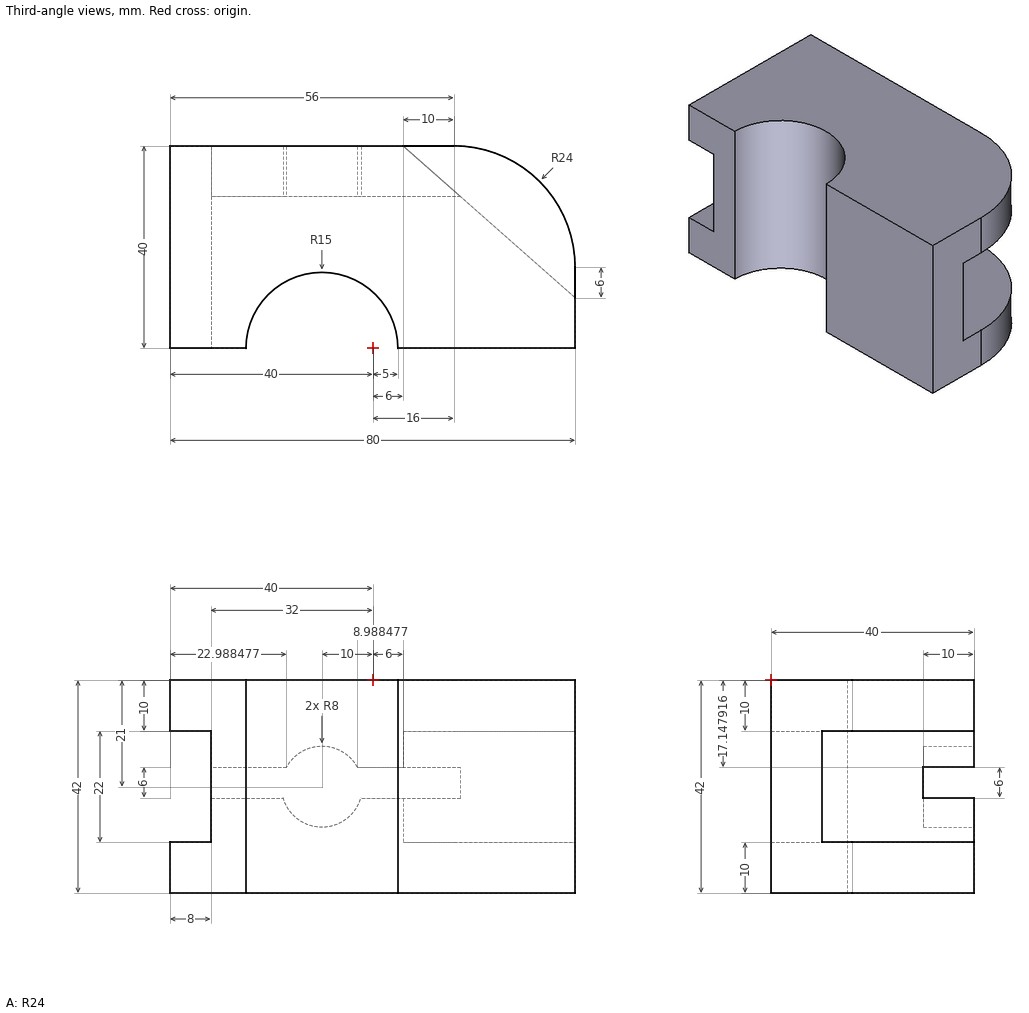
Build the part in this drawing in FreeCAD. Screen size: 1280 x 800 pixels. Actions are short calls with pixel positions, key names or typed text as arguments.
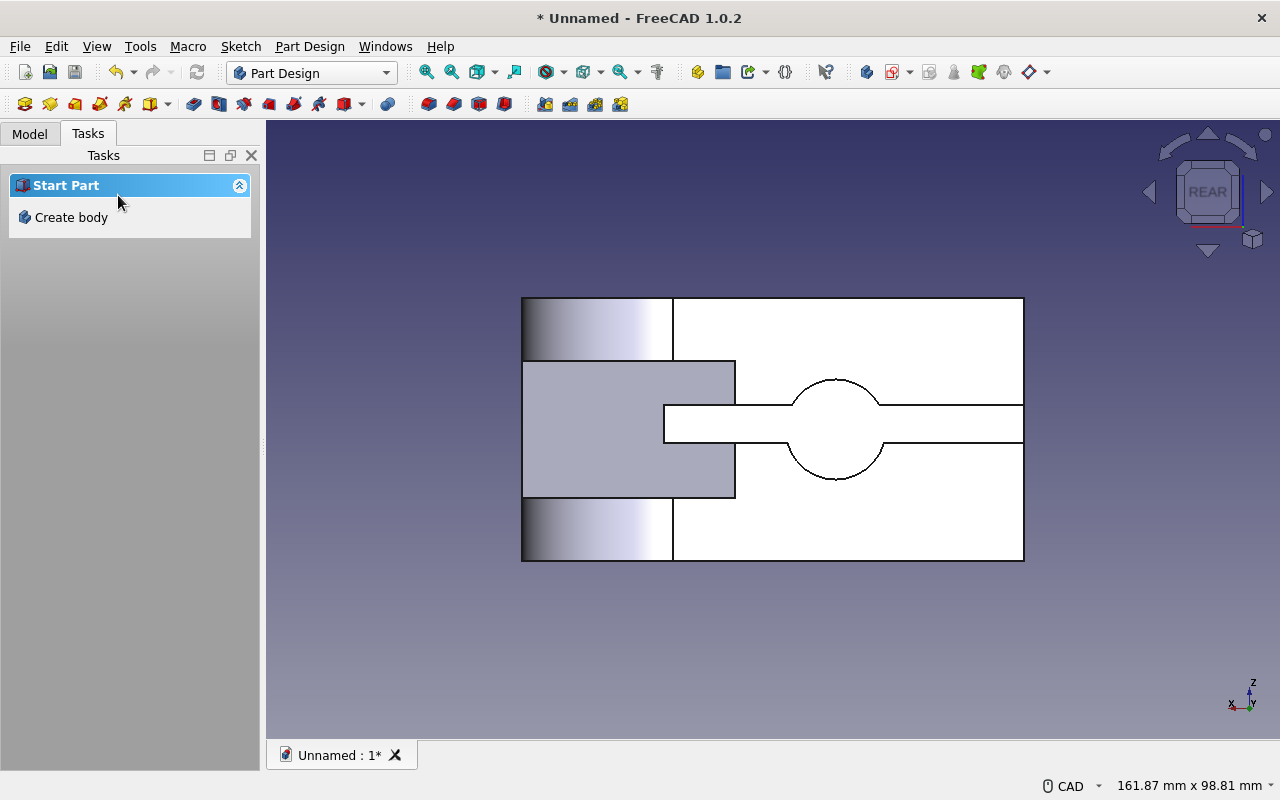
click(948, 501)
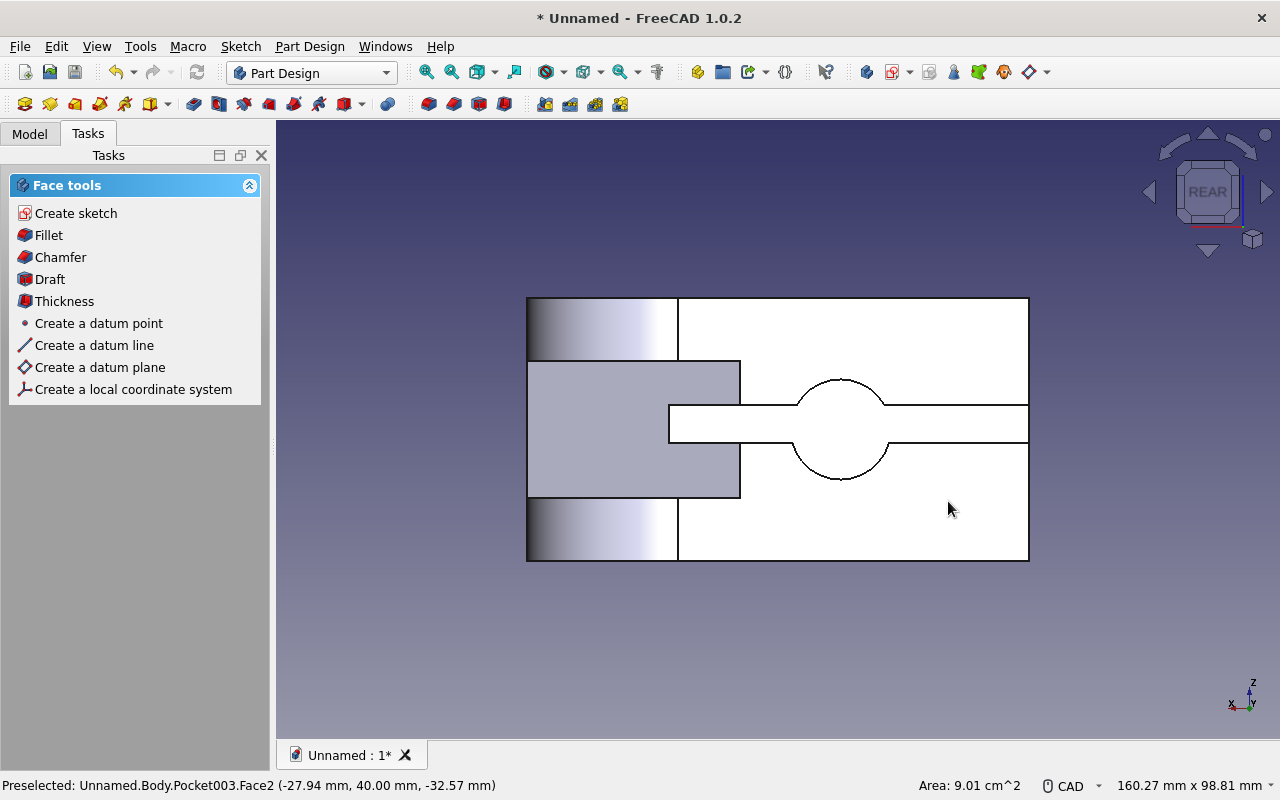
click(892, 72)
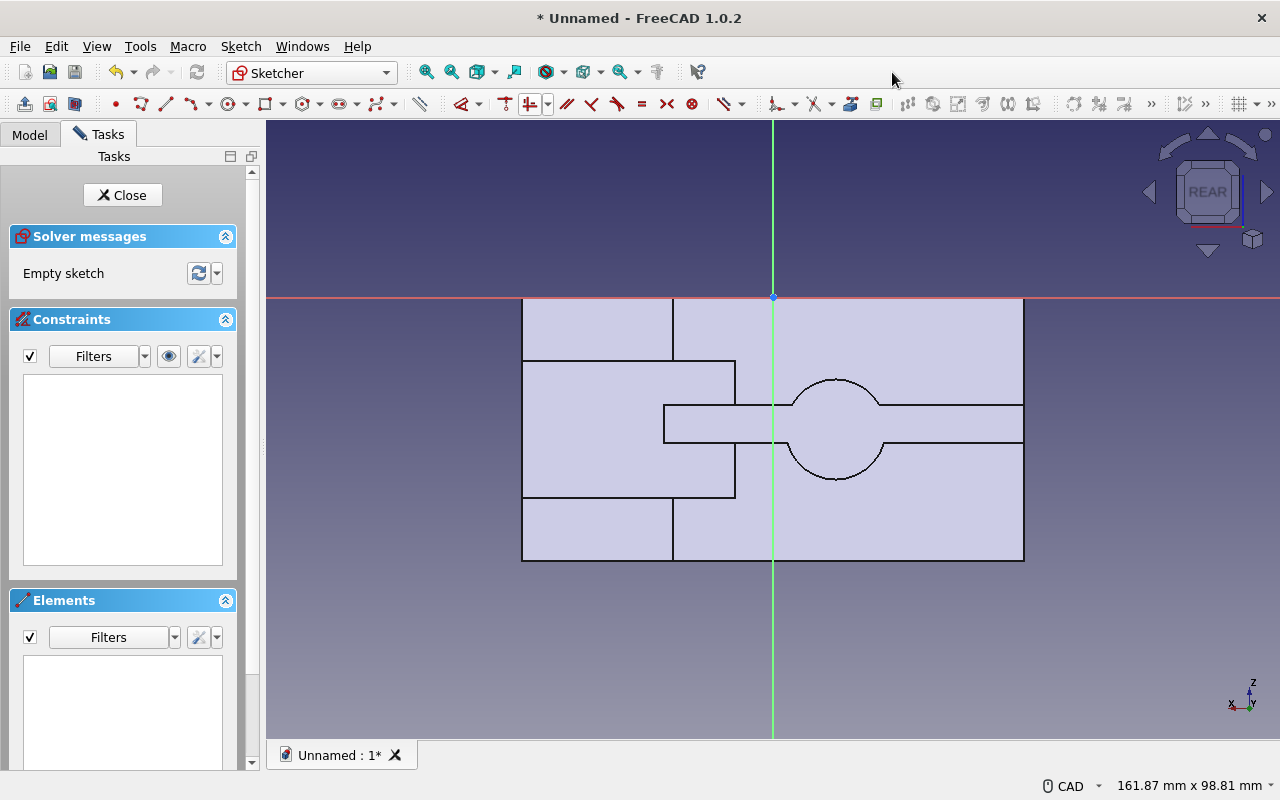
scroll(1115, 360, up, 3)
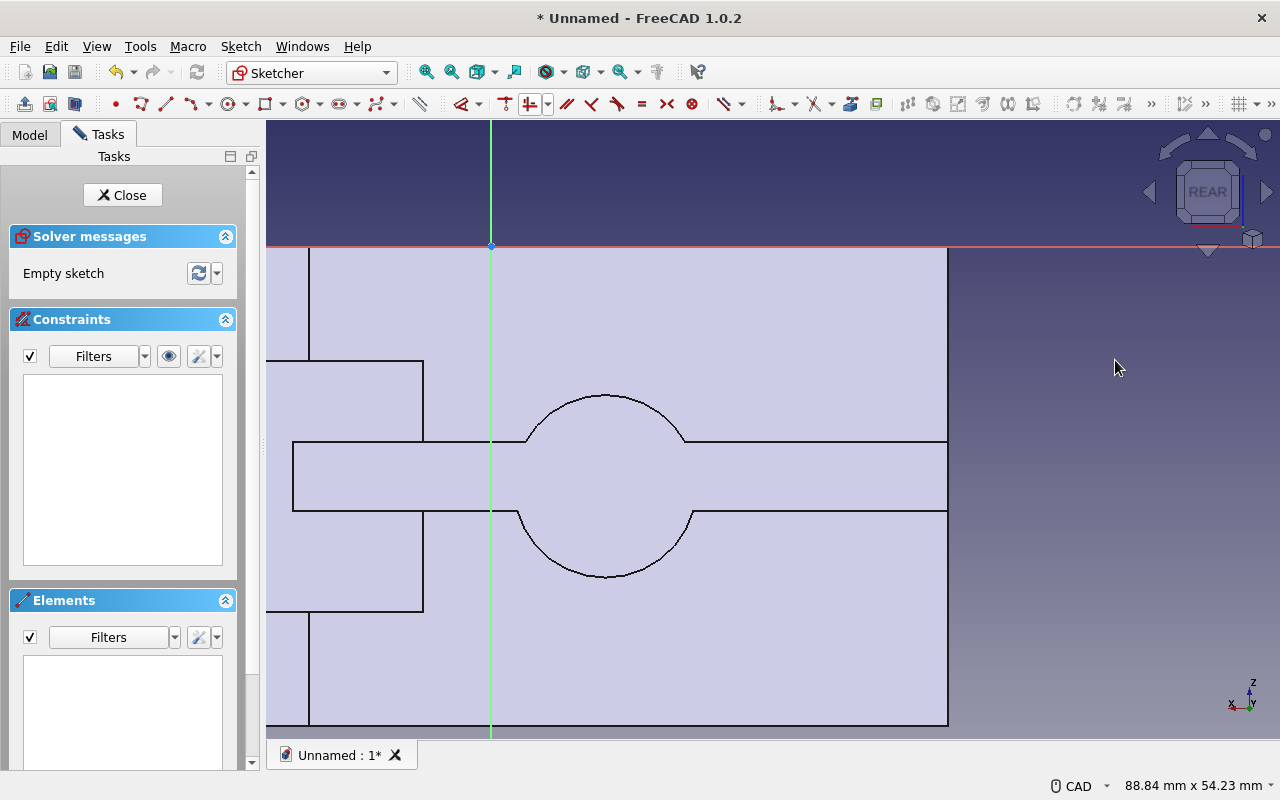
key(g)
key(r)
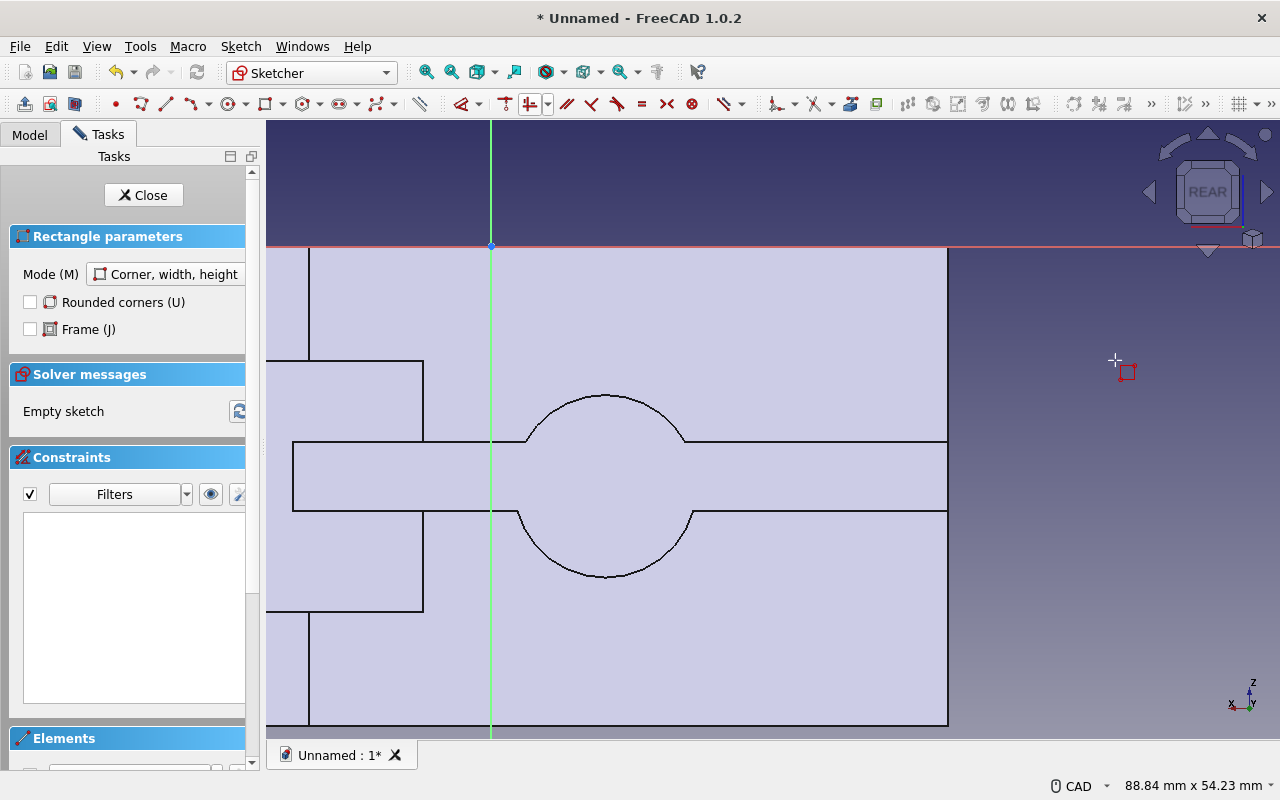
click(856, 361)
move(948, 612)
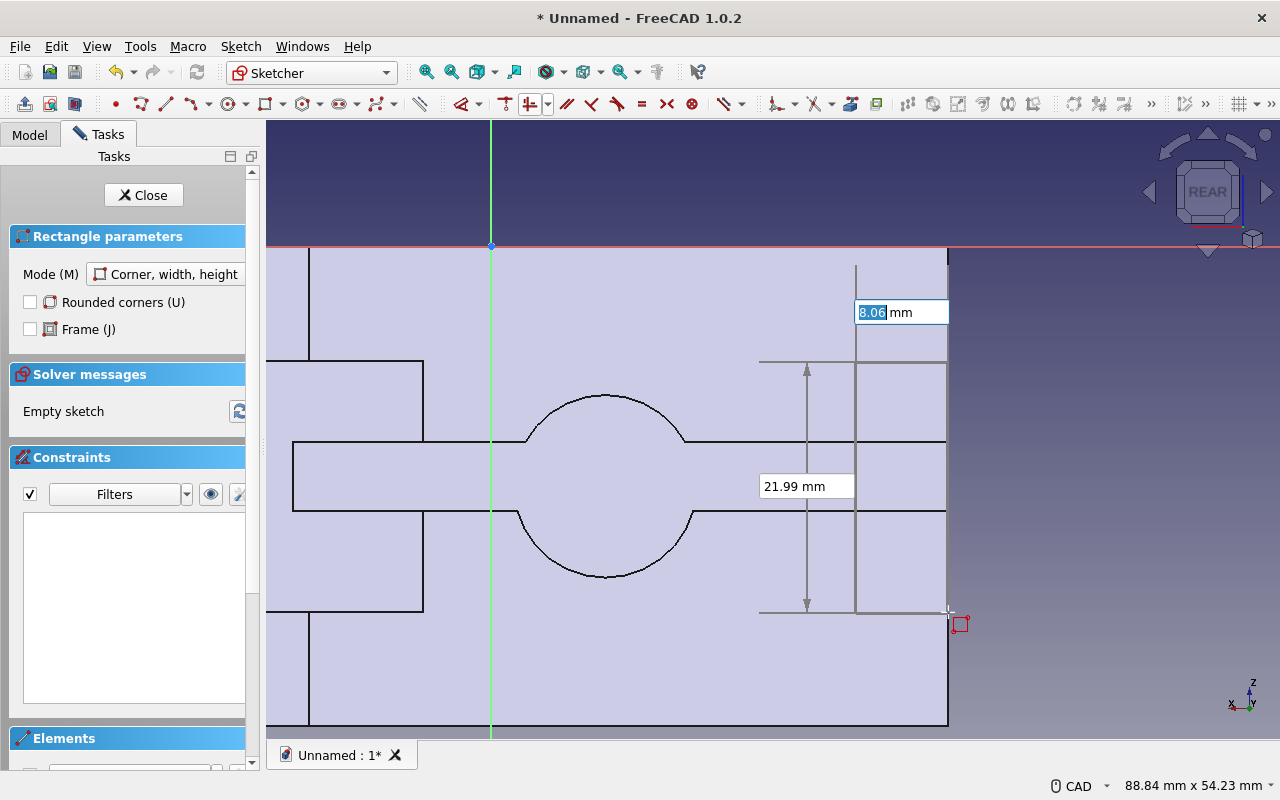
text(8)
key(Tab)
text(22)
key(Return)
key(Escape)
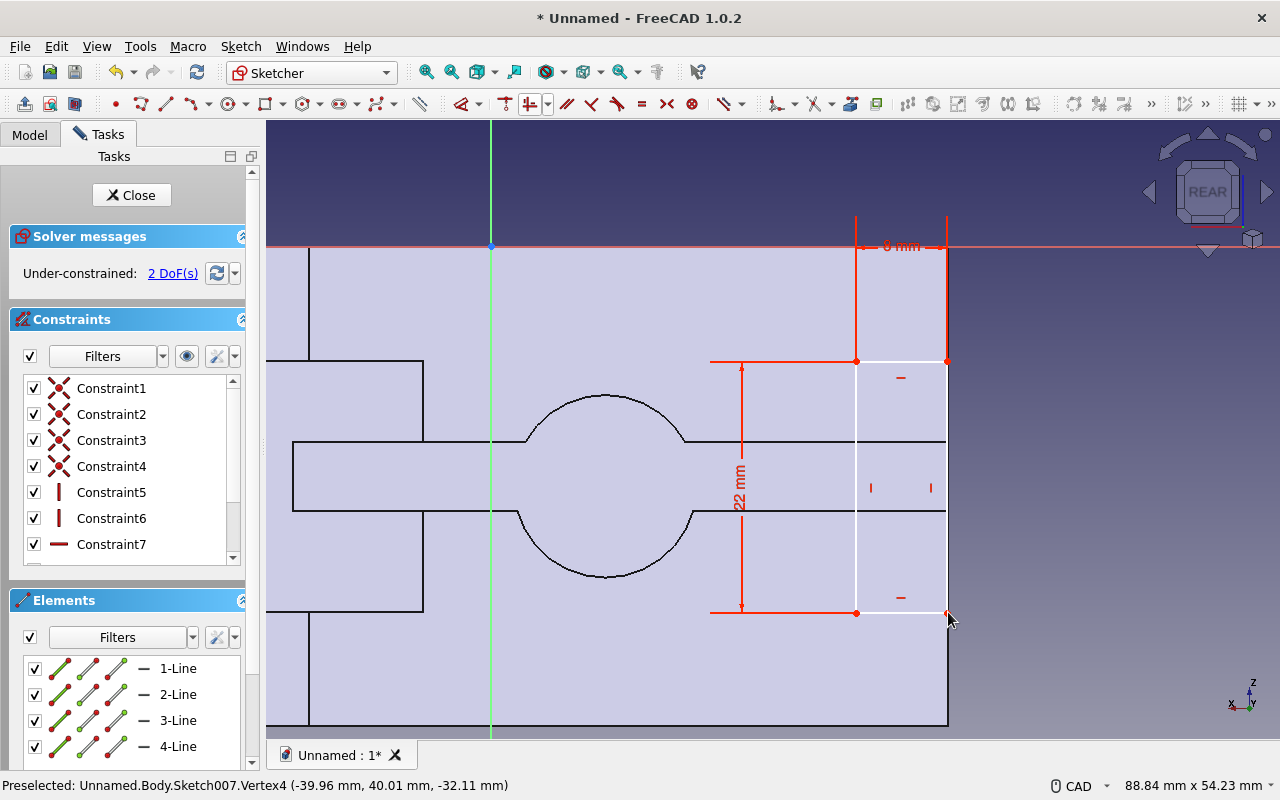
key(d)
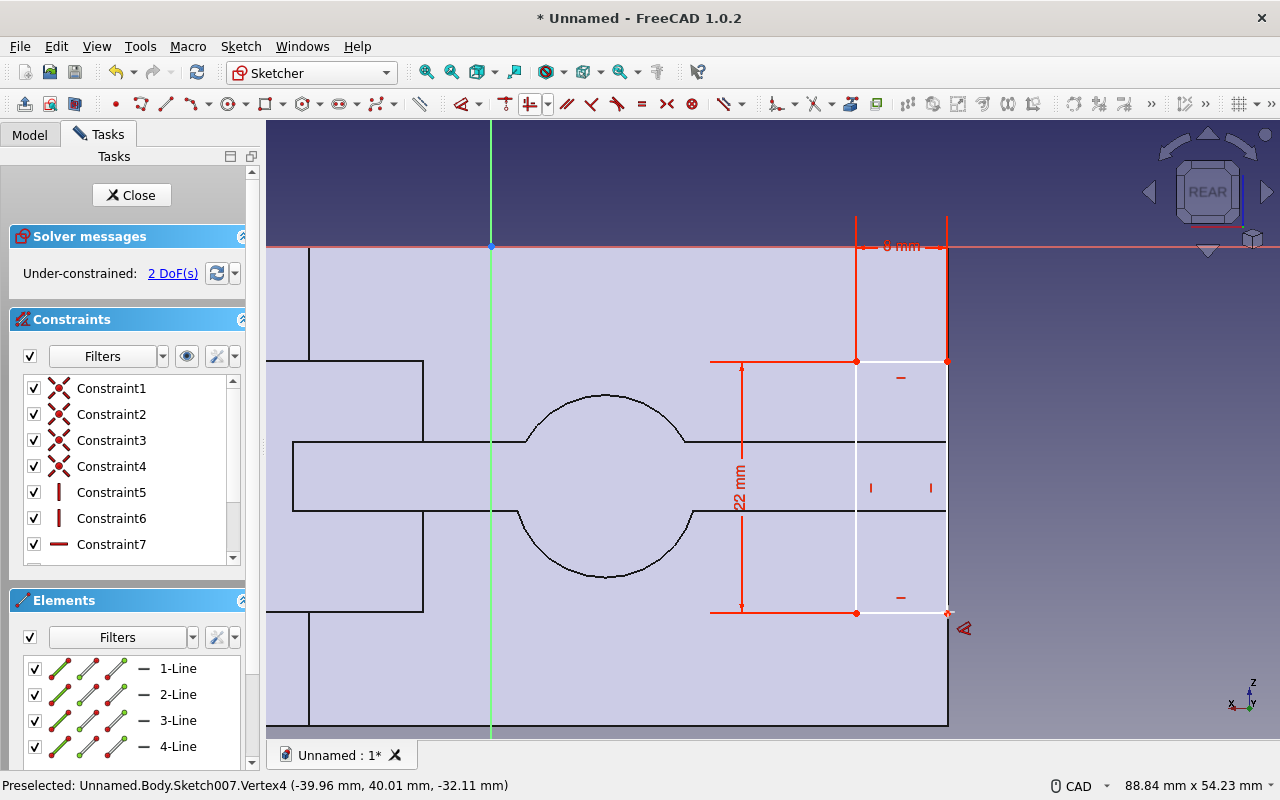
click(856, 362)
click(674, 213)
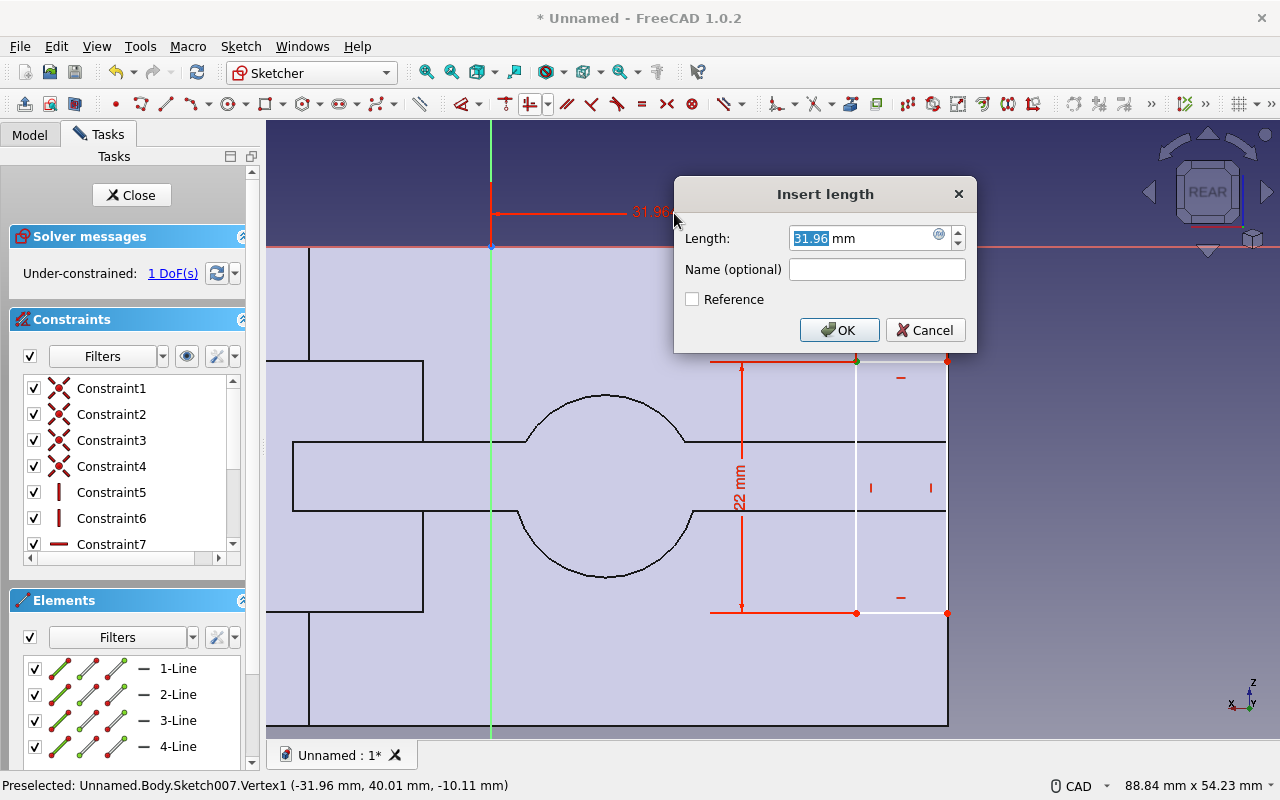
text(32)
key(Return)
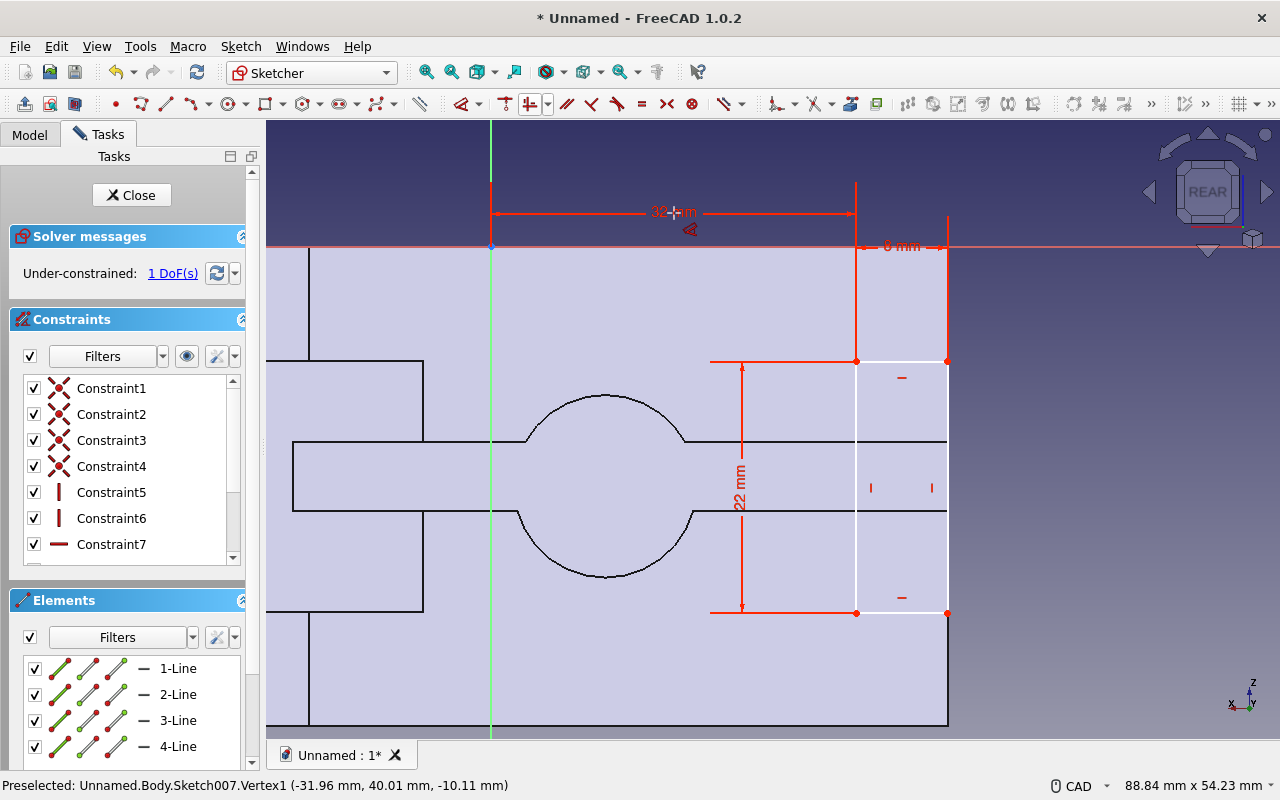
click(856, 362)
click(457, 304)